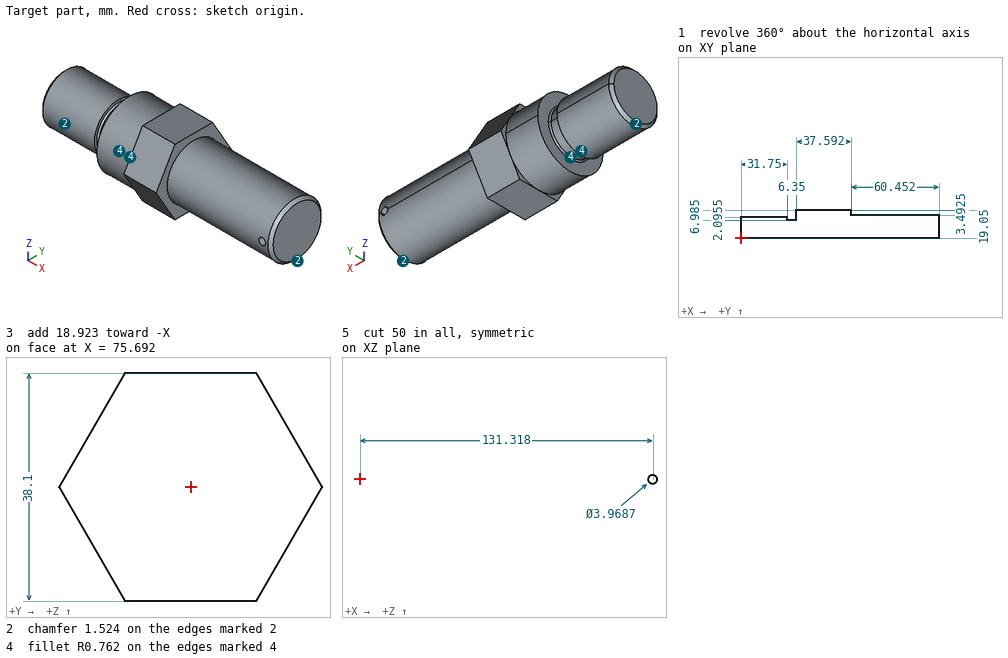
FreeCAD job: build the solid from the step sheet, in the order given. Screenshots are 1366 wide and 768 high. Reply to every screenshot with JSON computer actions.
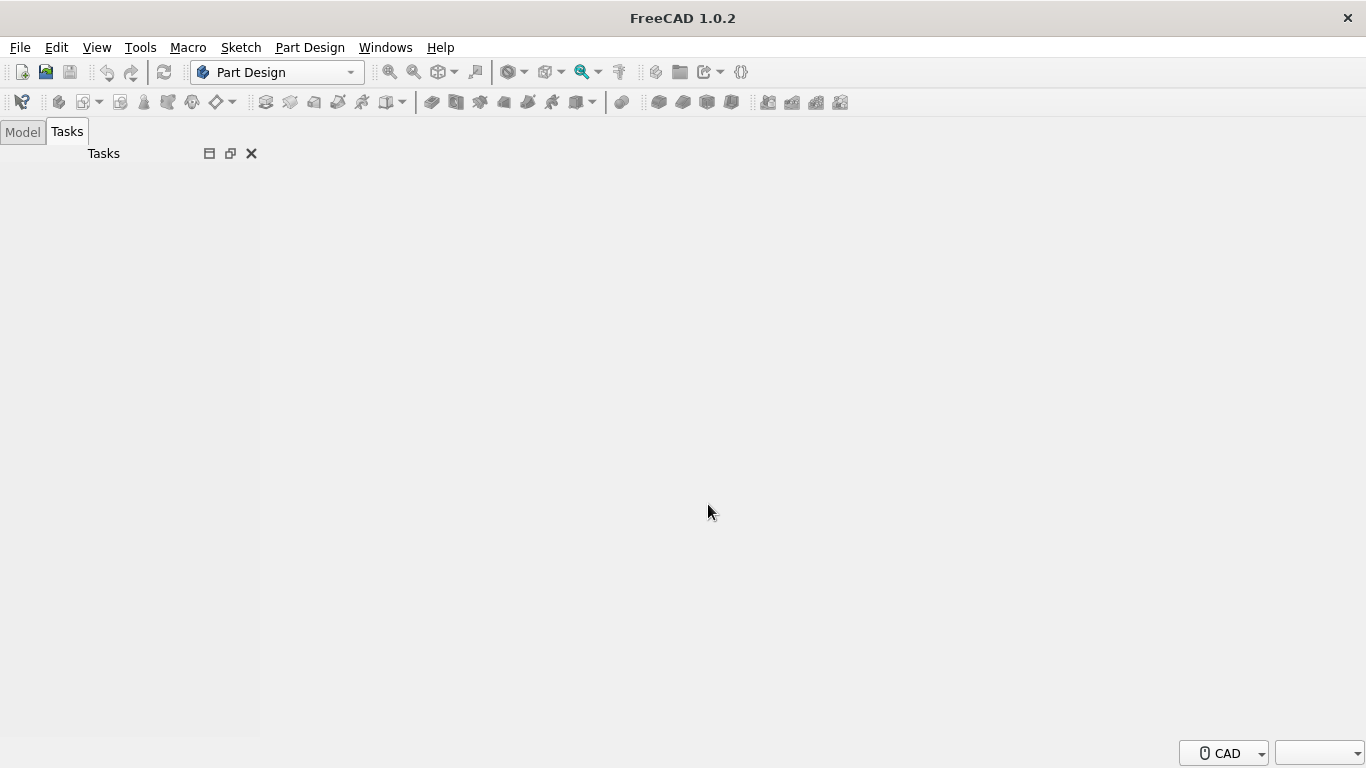
{"action": "key", "text": "ctrl+n"}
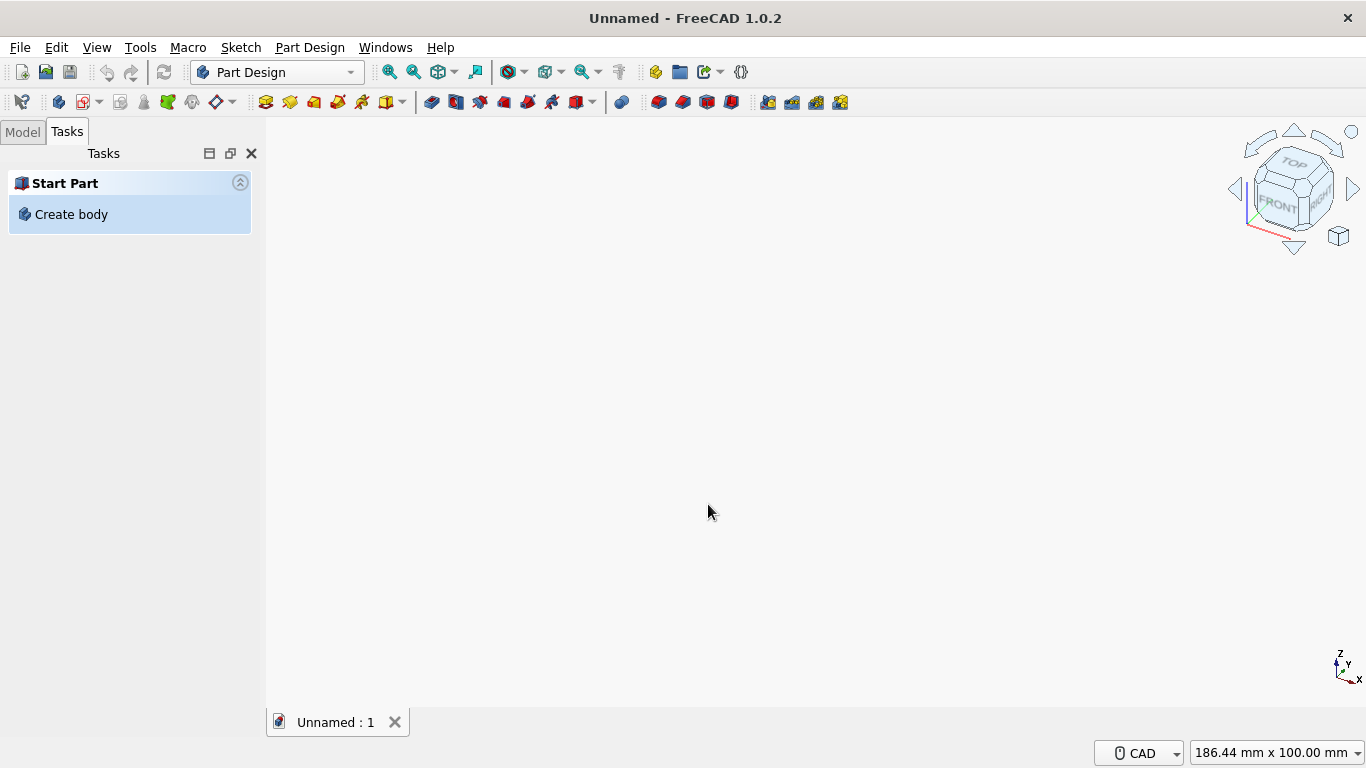
{"action": "left_click", "coordinate": [84, 102]}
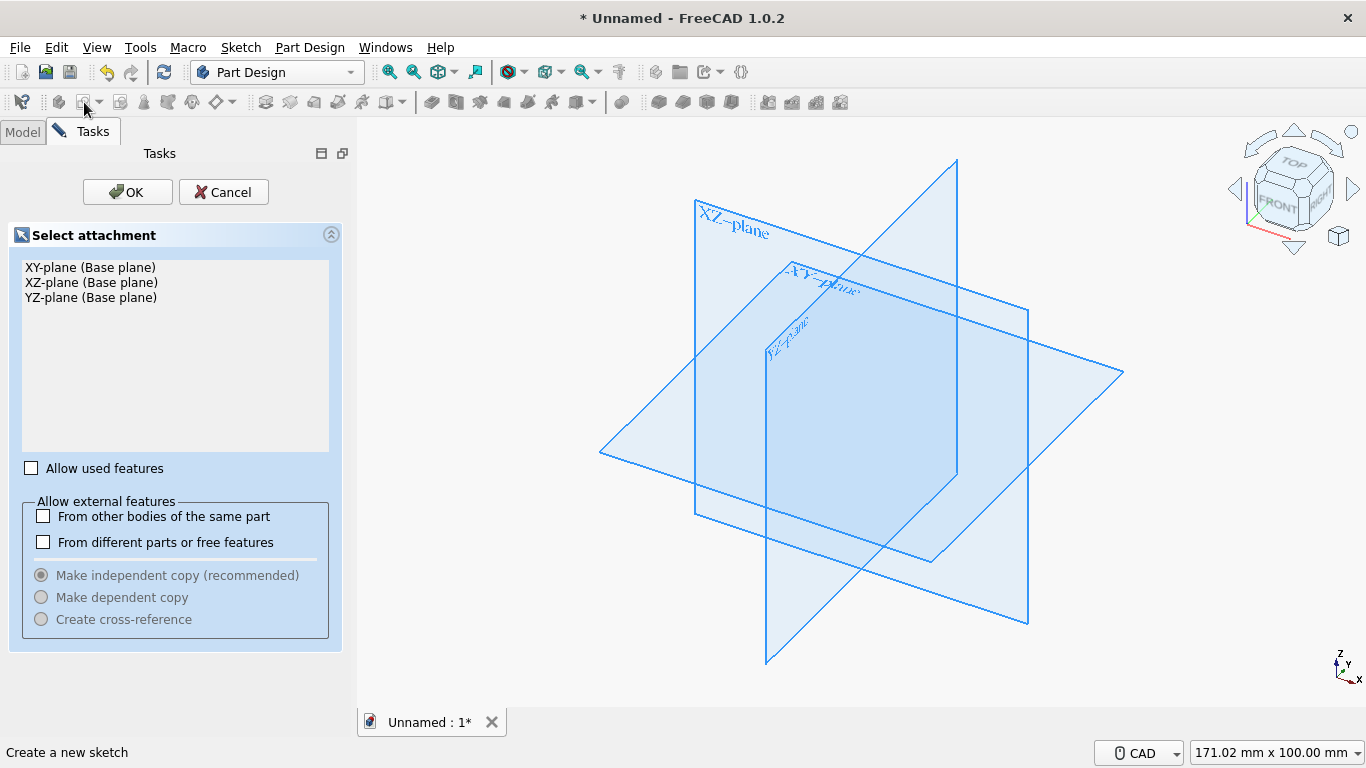
{"action": "left_click", "coordinate": [82, 268]}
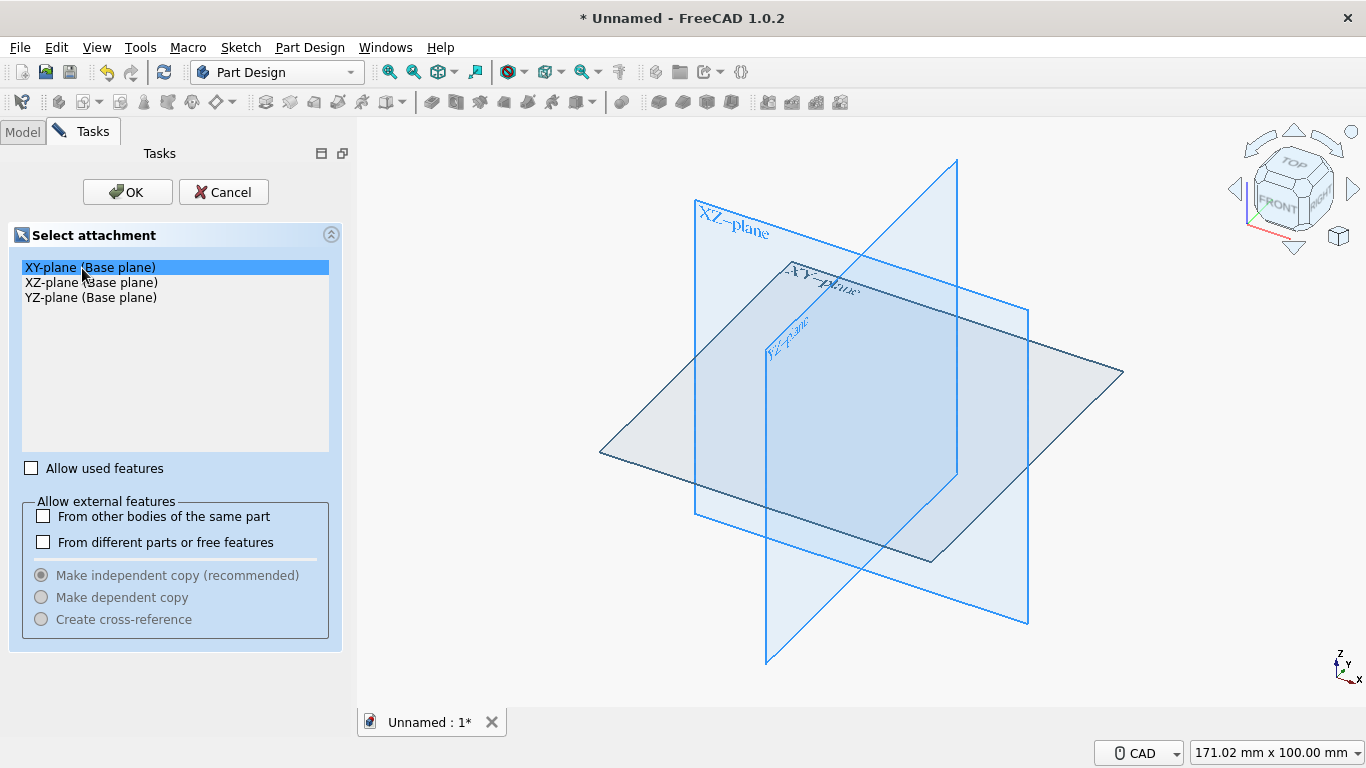
{"action": "left_click", "coordinate": [128, 192]}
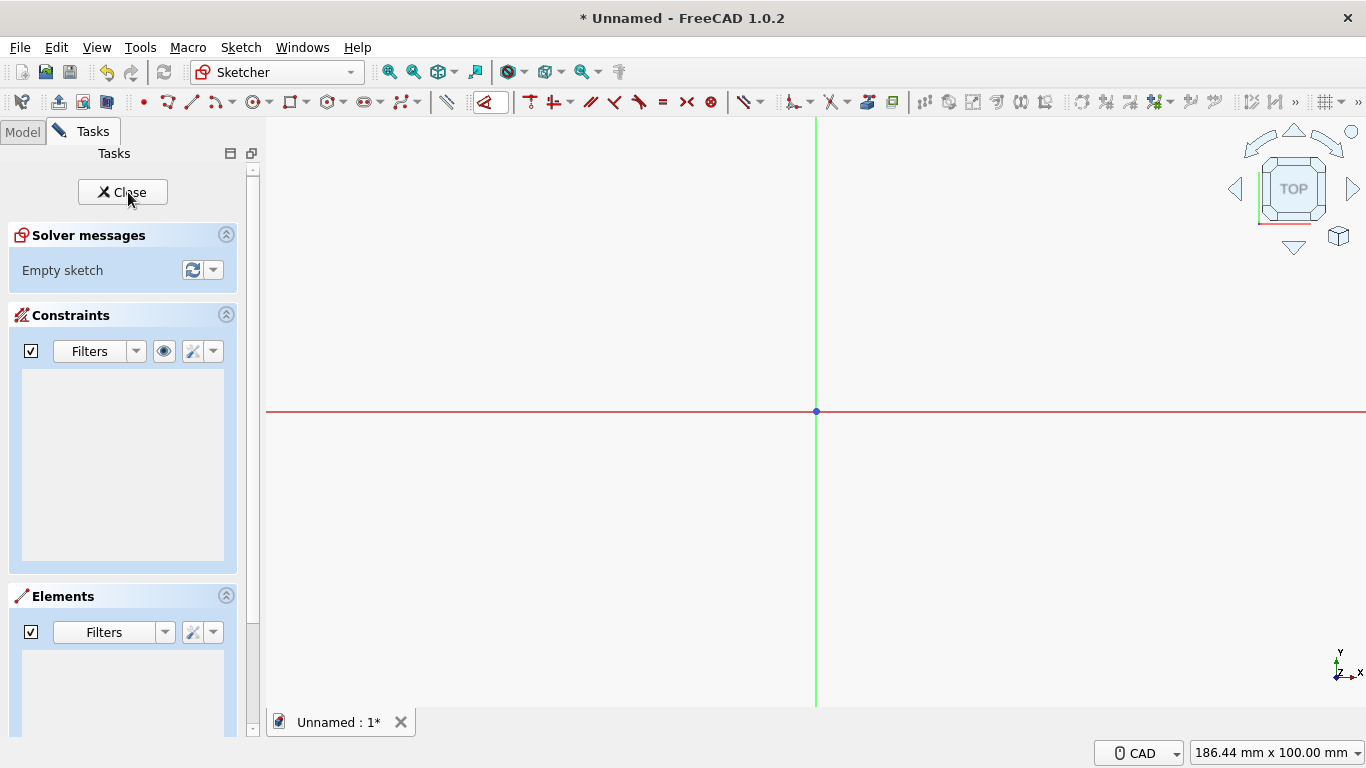
{"action": "scroll", "coordinate": [294, 480], "scroll_direction": "down", "scroll_amount": 3}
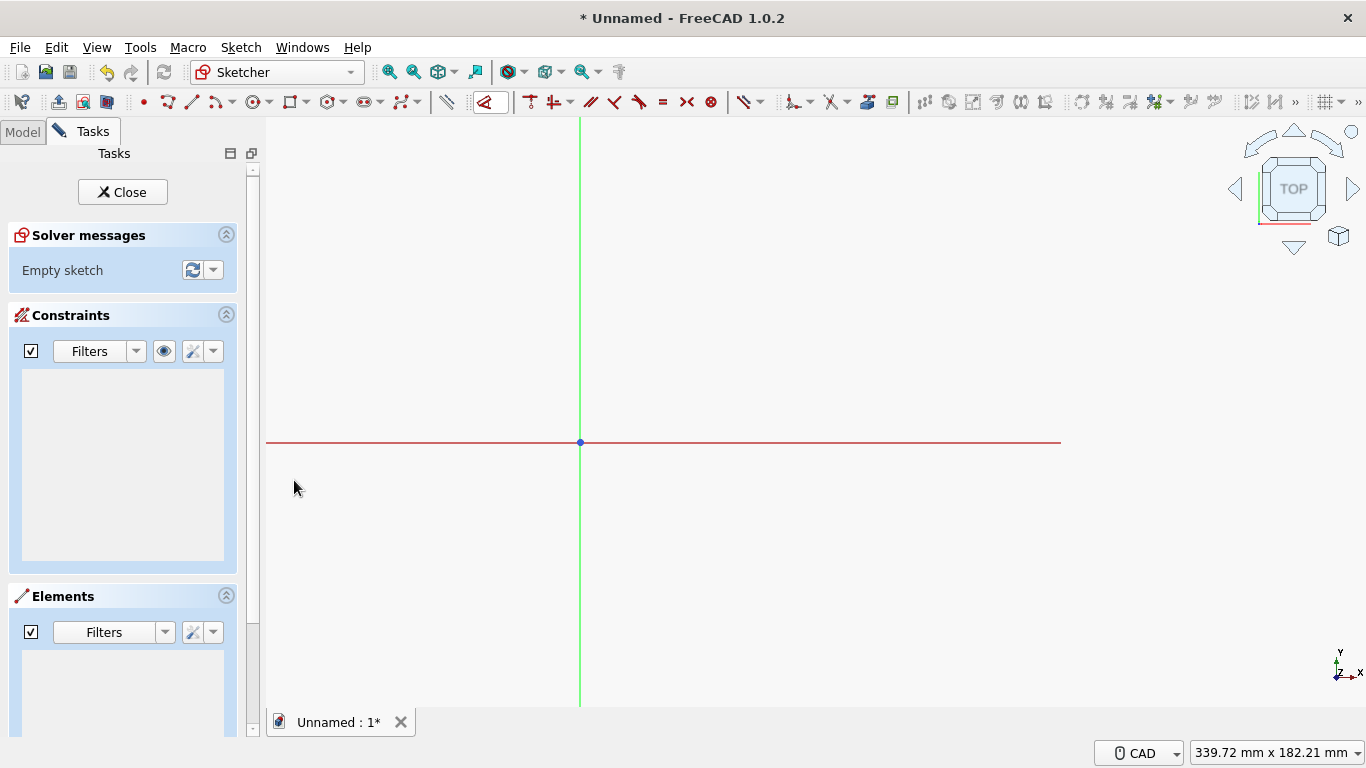
{"action": "scroll", "coordinate": [909, 412], "scroll_direction": "up", "scroll_amount": 2}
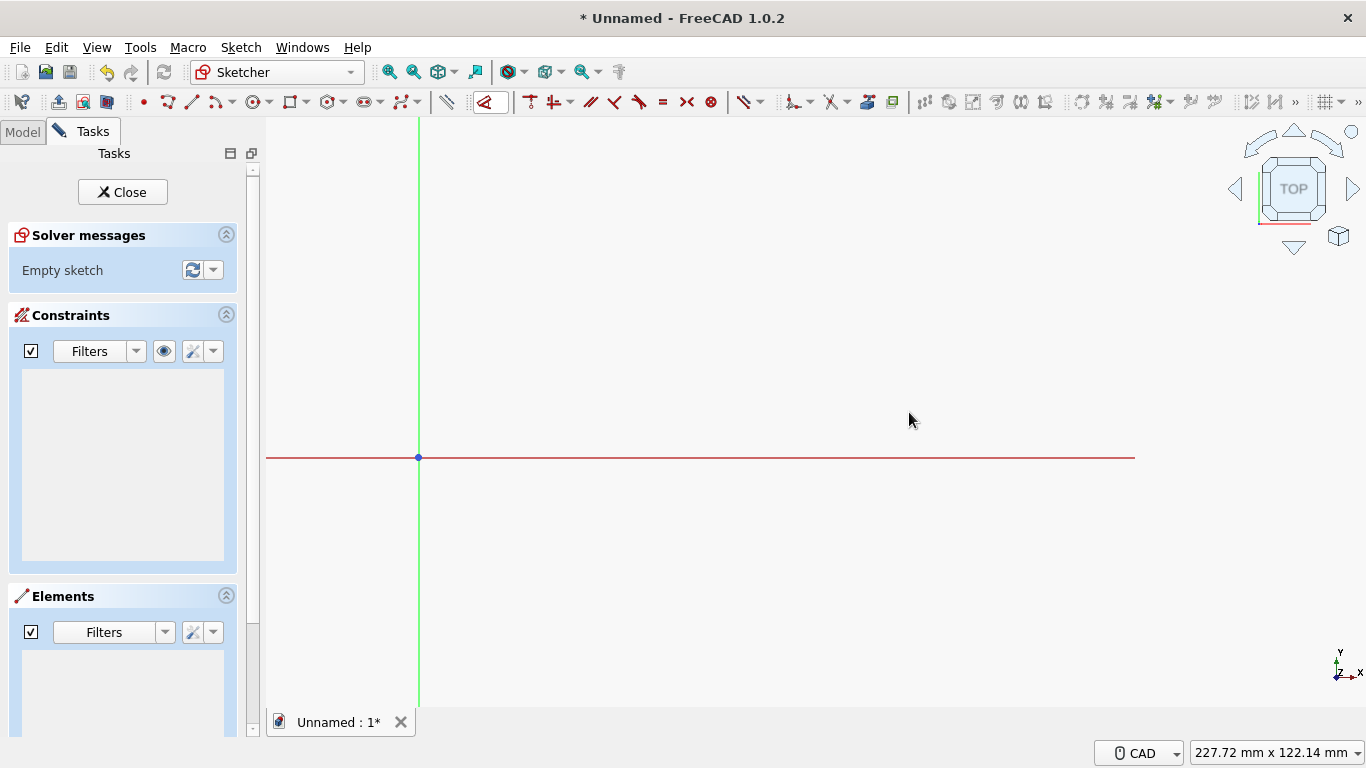
{"action": "key", "text": "g m"}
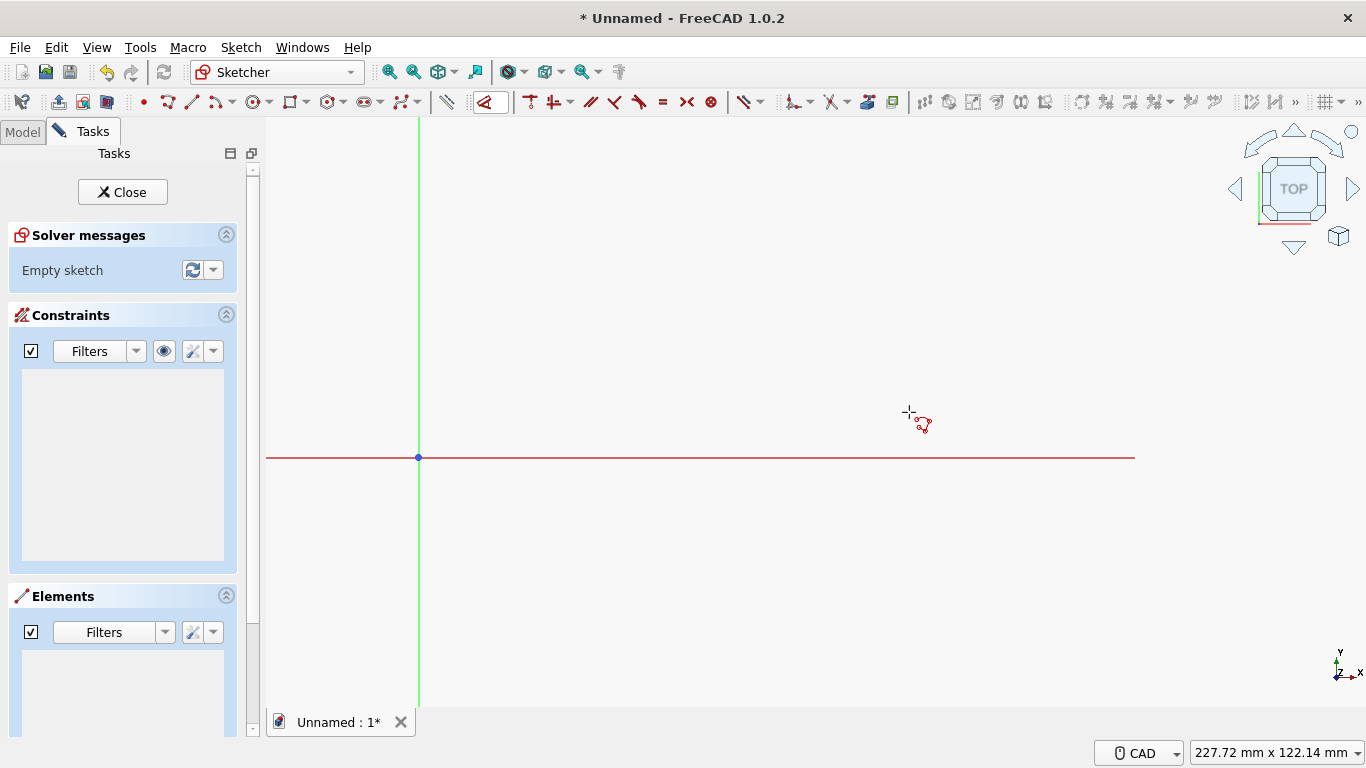
{"action": "left_click", "coordinate": [419, 458]}
{"action": "left_click", "coordinate": [1076, 449]}
{"action": "left_click", "coordinate": [1076, 383]}
{"action": "left_click", "coordinate": [784, 383]}
{"action": "left_click", "coordinate": [784, 366]}
{"action": "left_click", "coordinate": [603, 366]}
{"action": "left_click", "coordinate": [603, 400]}
{"action": "left_click", "coordinate": [572, 400]}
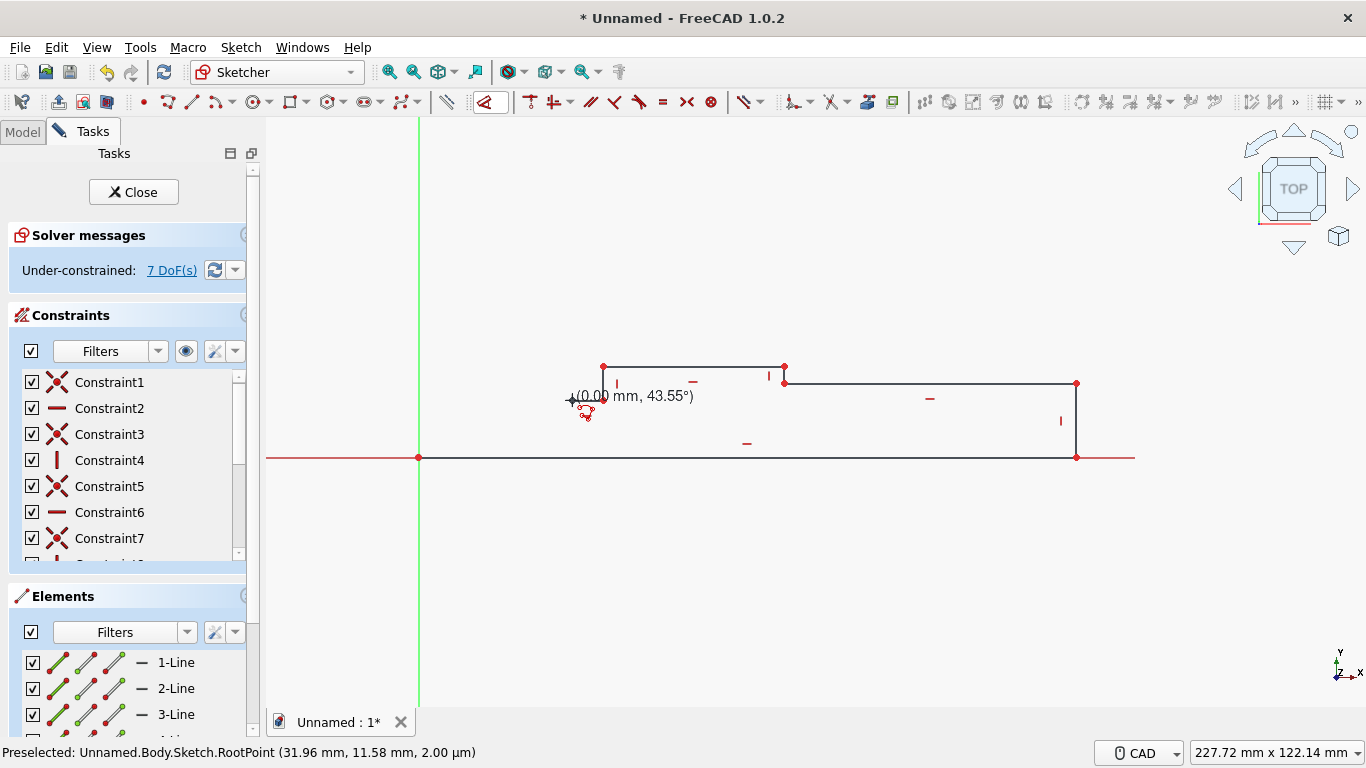
{"action": "scroll", "coordinate": [572, 390], "scroll_direction": "up", "scroll_amount": 3}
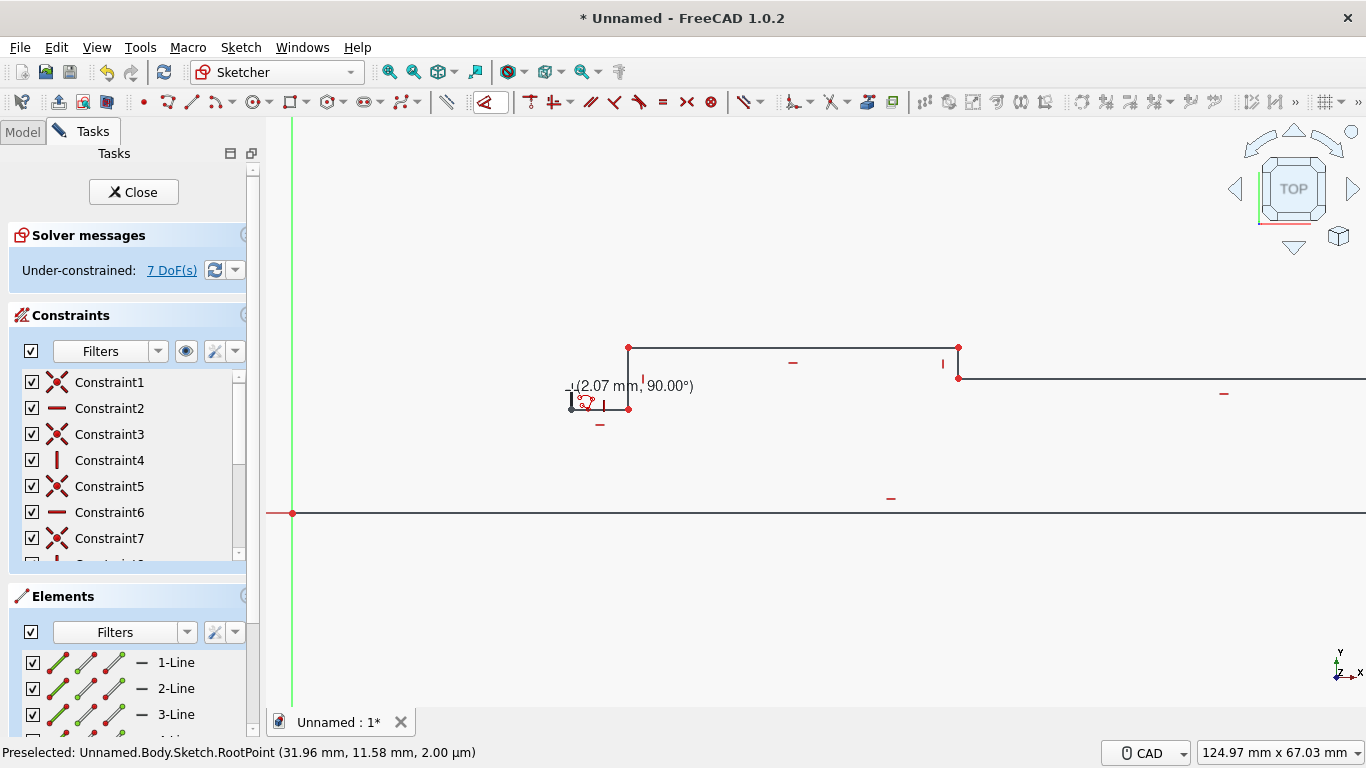
{"action": "left_click", "coordinate": [572, 389]}